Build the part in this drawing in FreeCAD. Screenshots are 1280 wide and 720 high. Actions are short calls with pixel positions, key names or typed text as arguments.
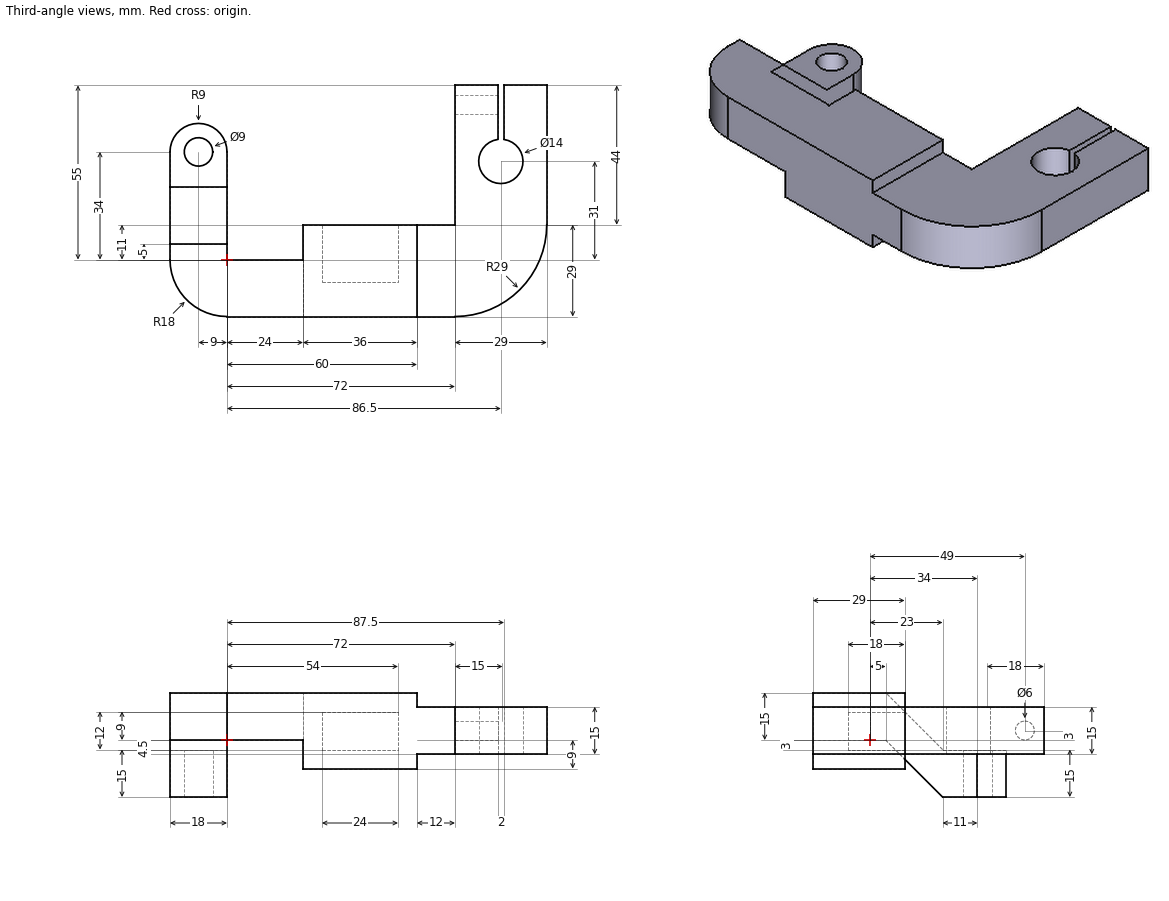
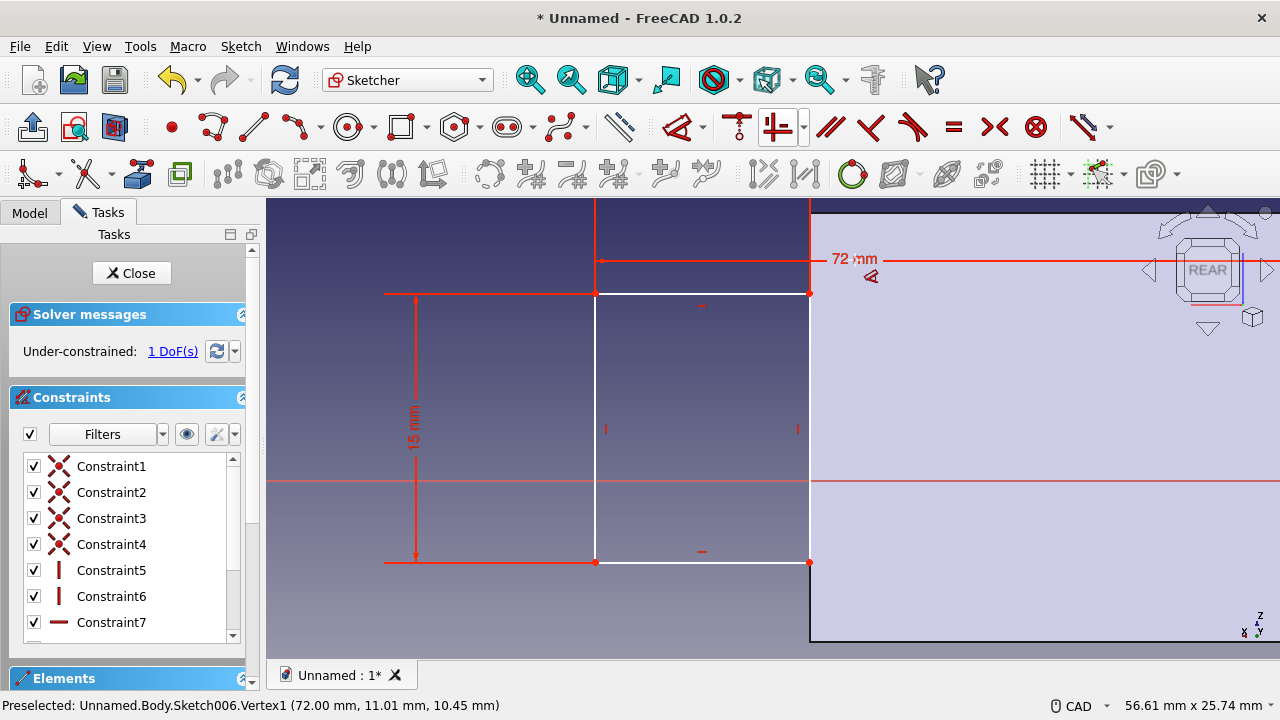
click(595, 563)
click(561, 522)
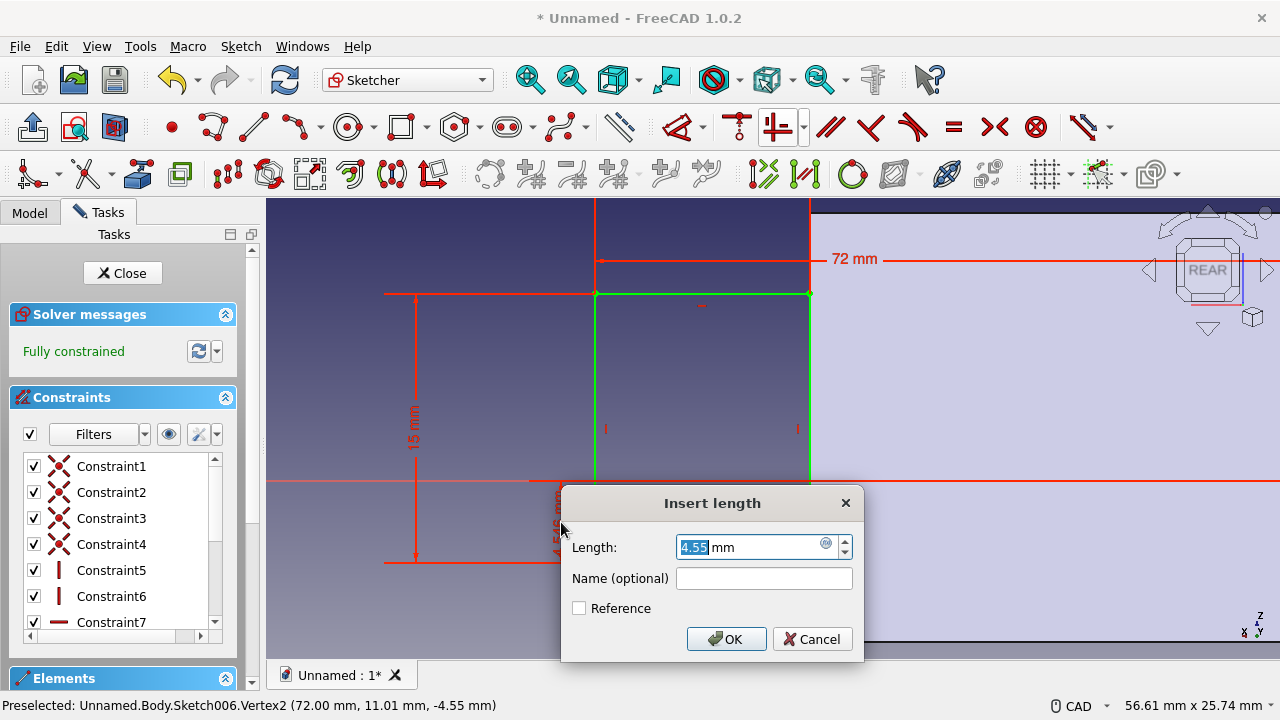
text(4.5)
key(Return)
key(Escape)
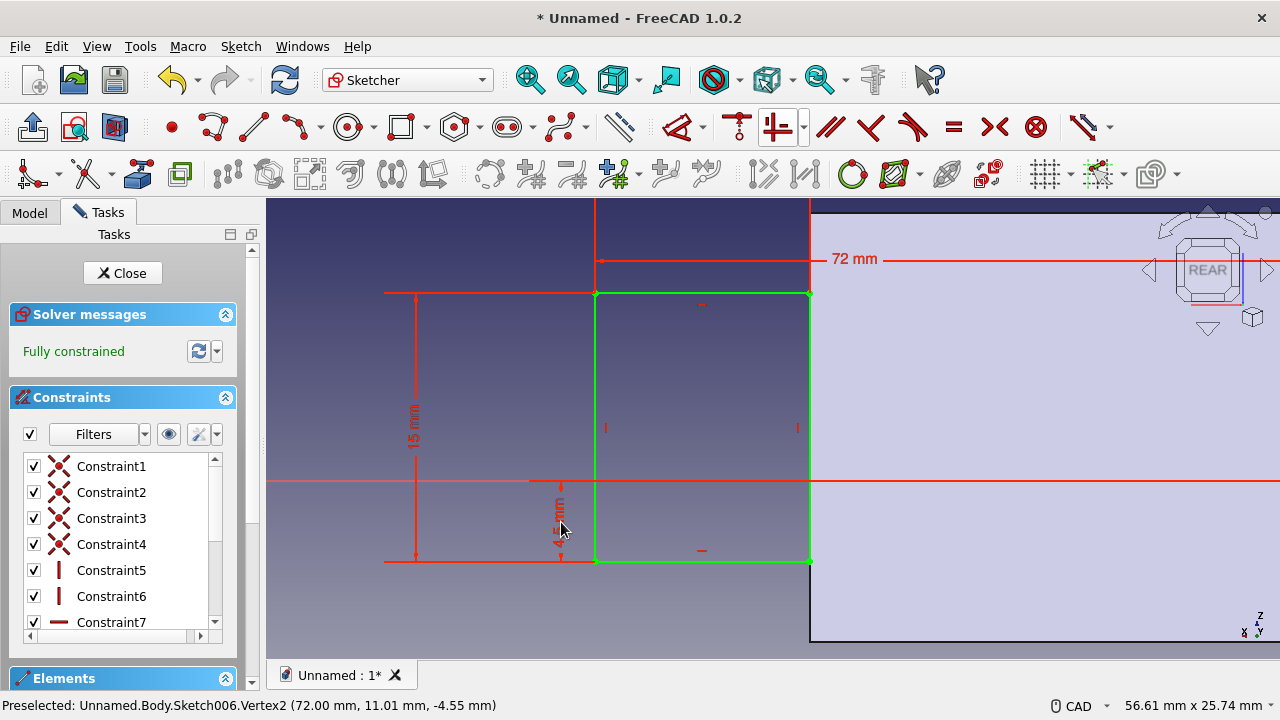
click(123, 273)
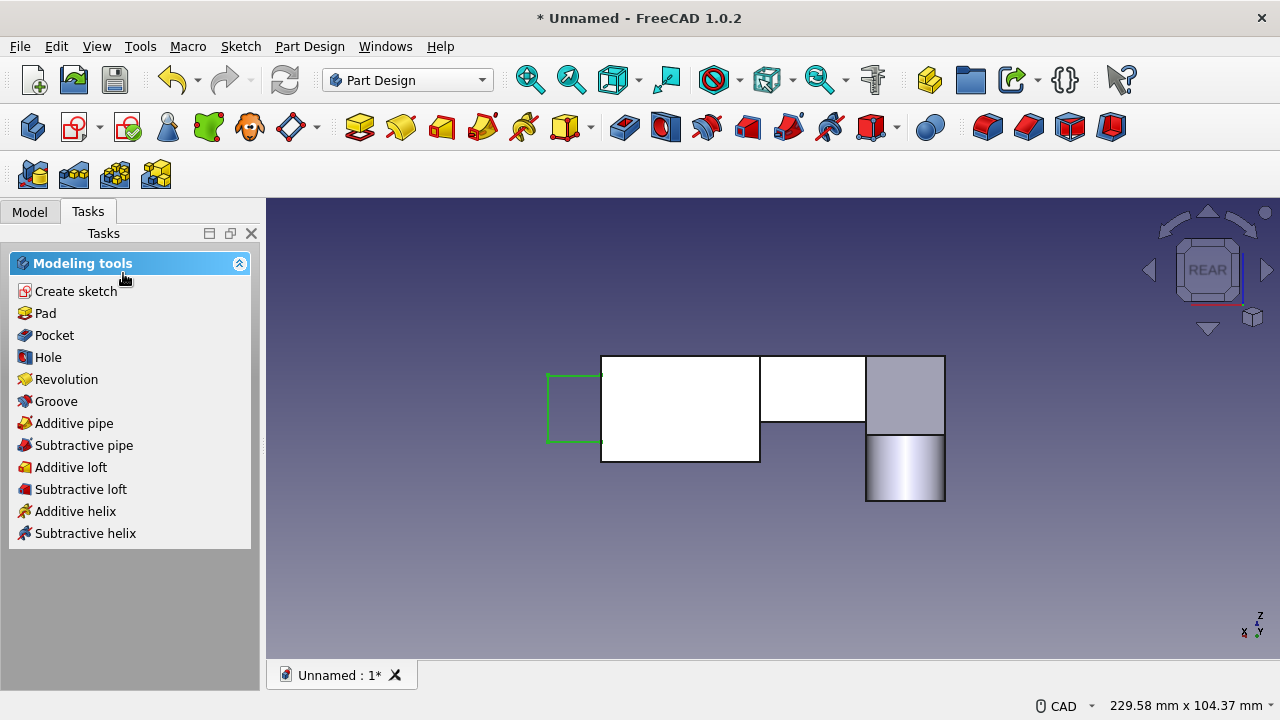
click(360, 128)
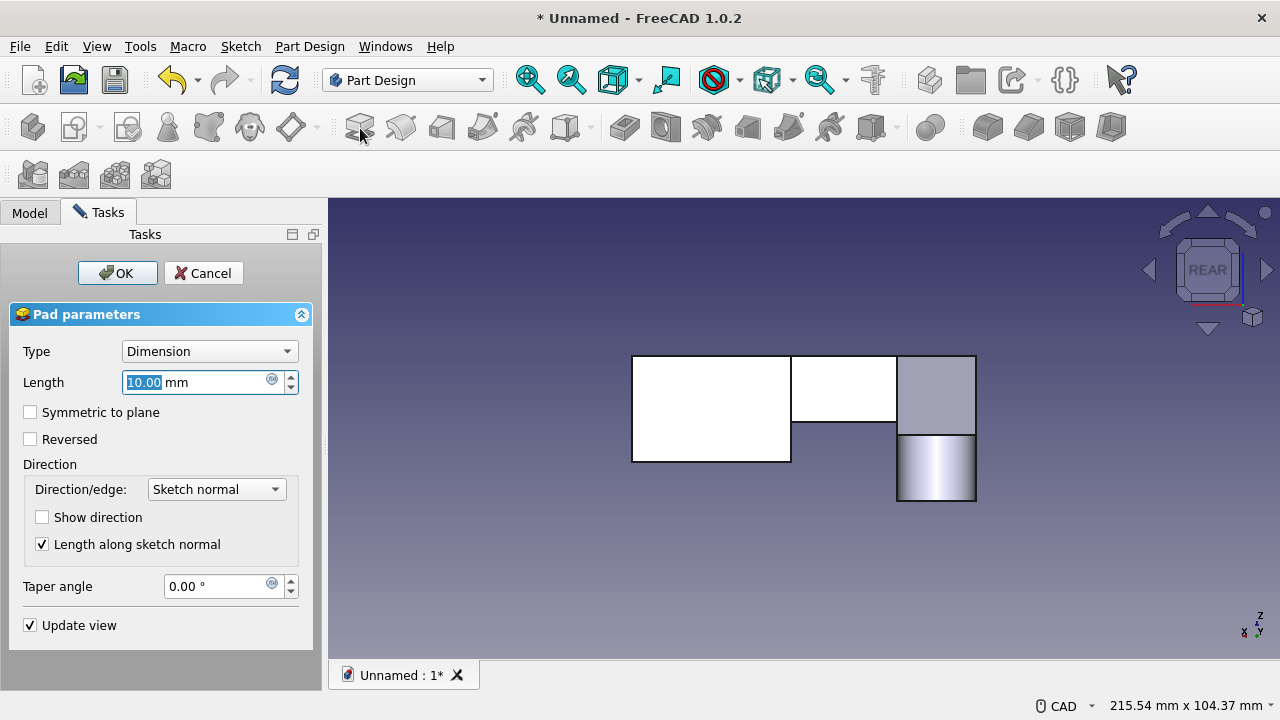
text(29)
key(Tab)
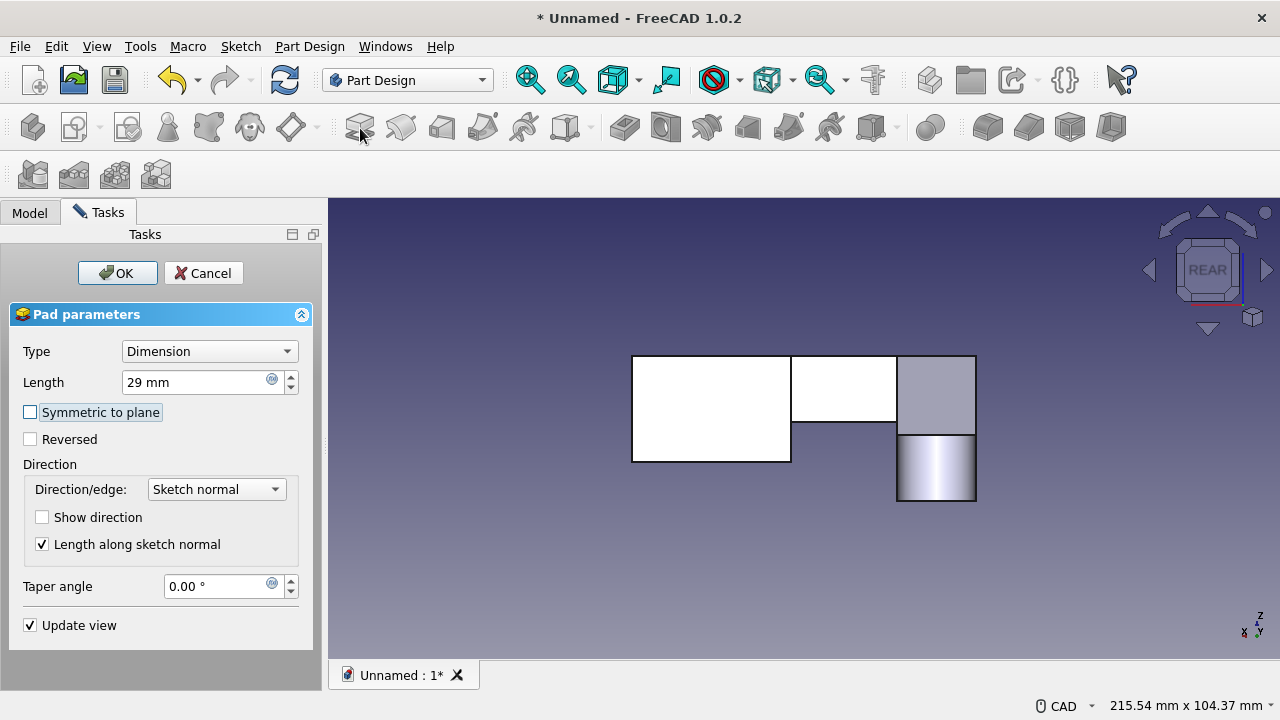
click(31, 439)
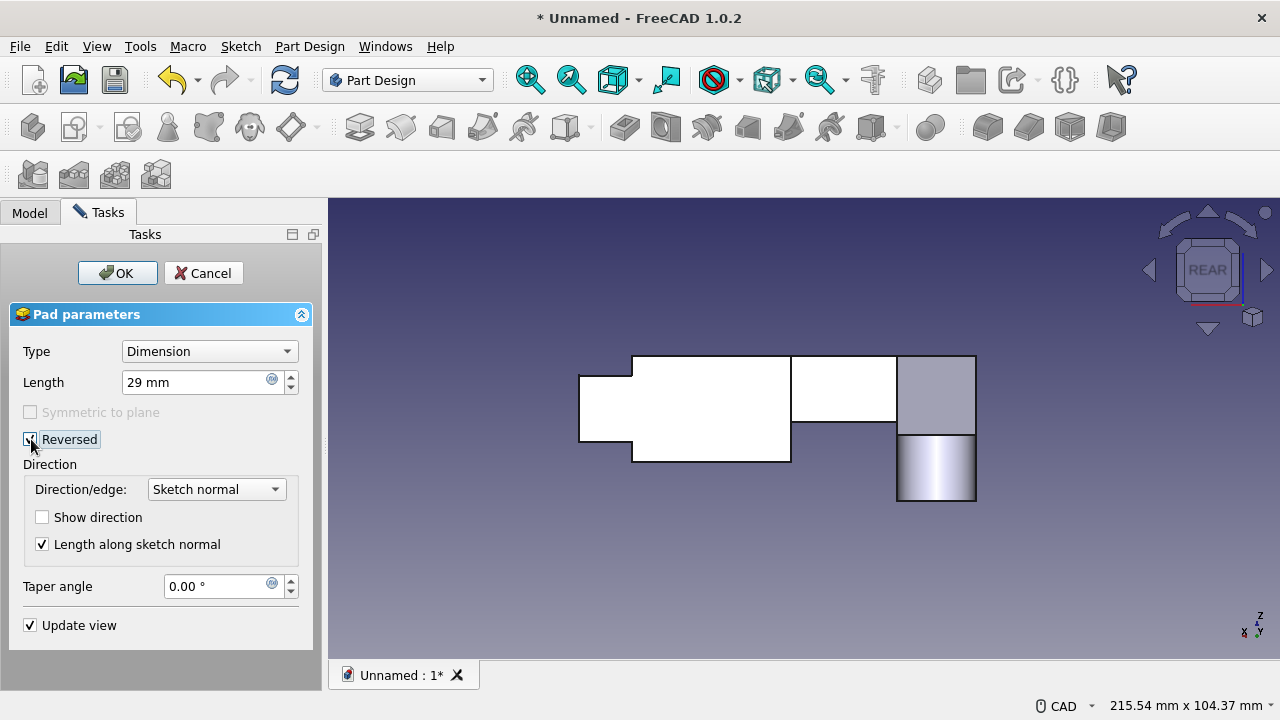
click(118, 273)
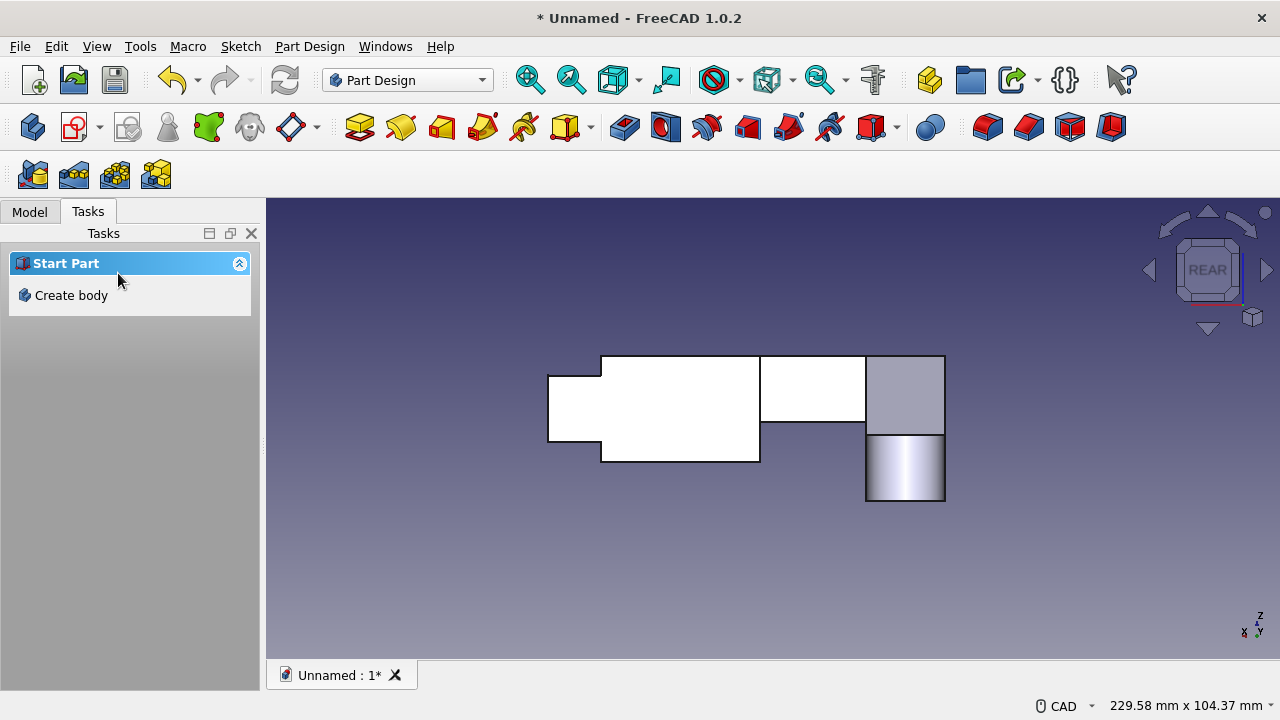
click(531, 80)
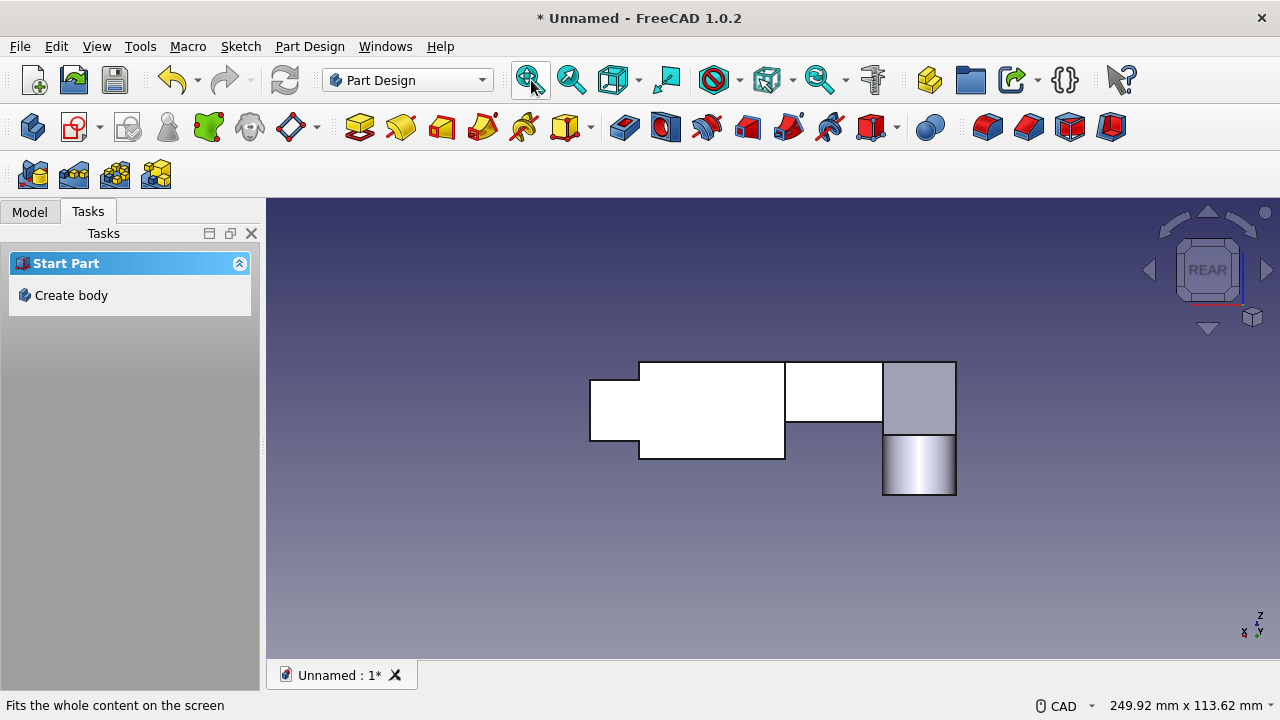
key(0)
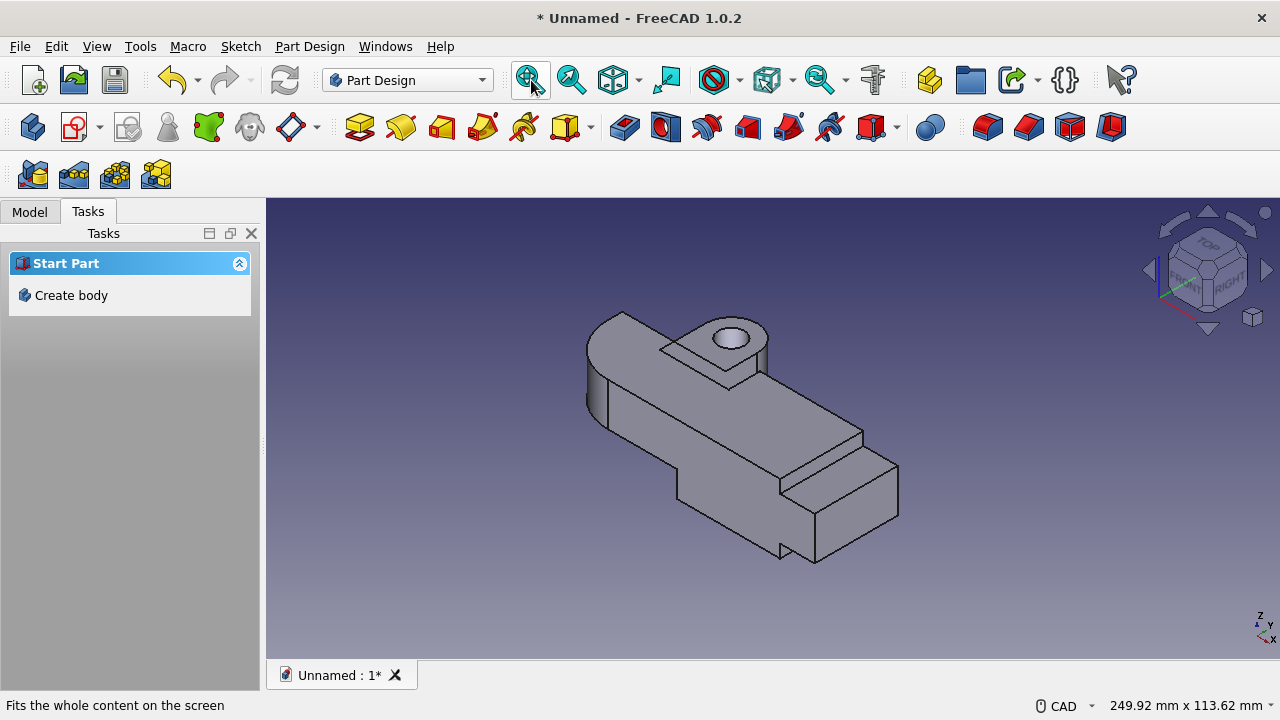
click(863, 465)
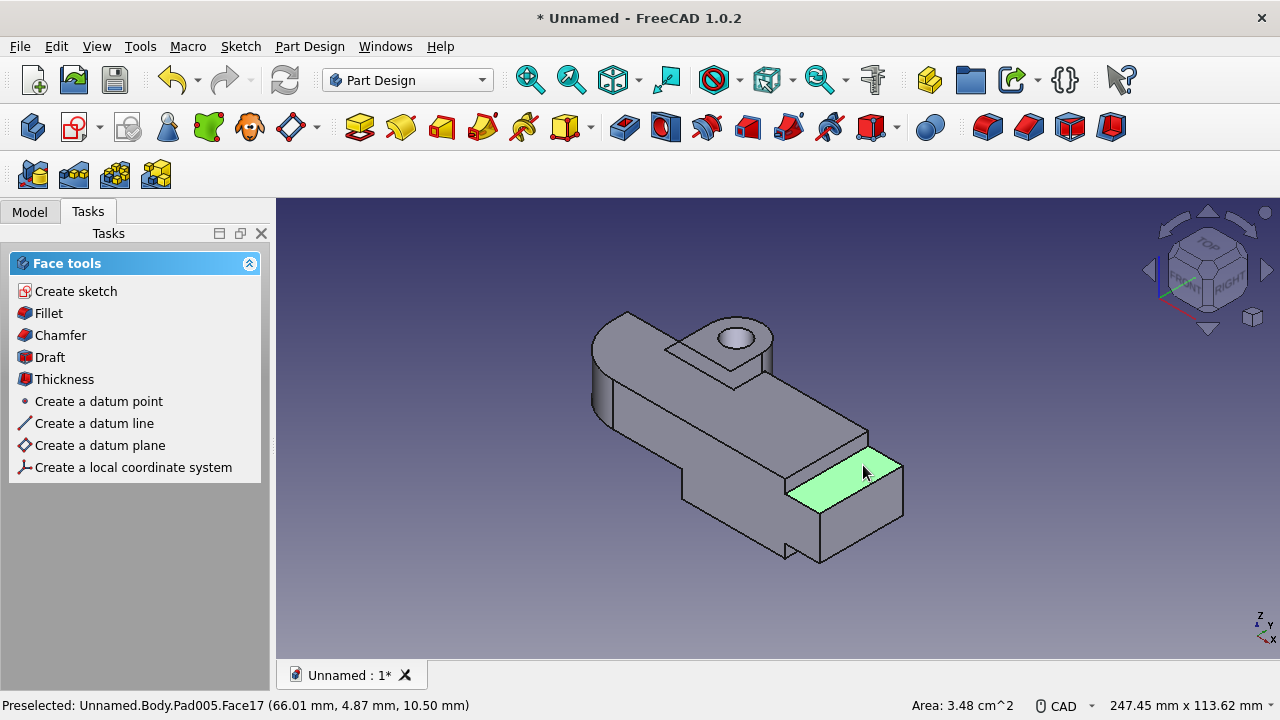
click(74, 128)